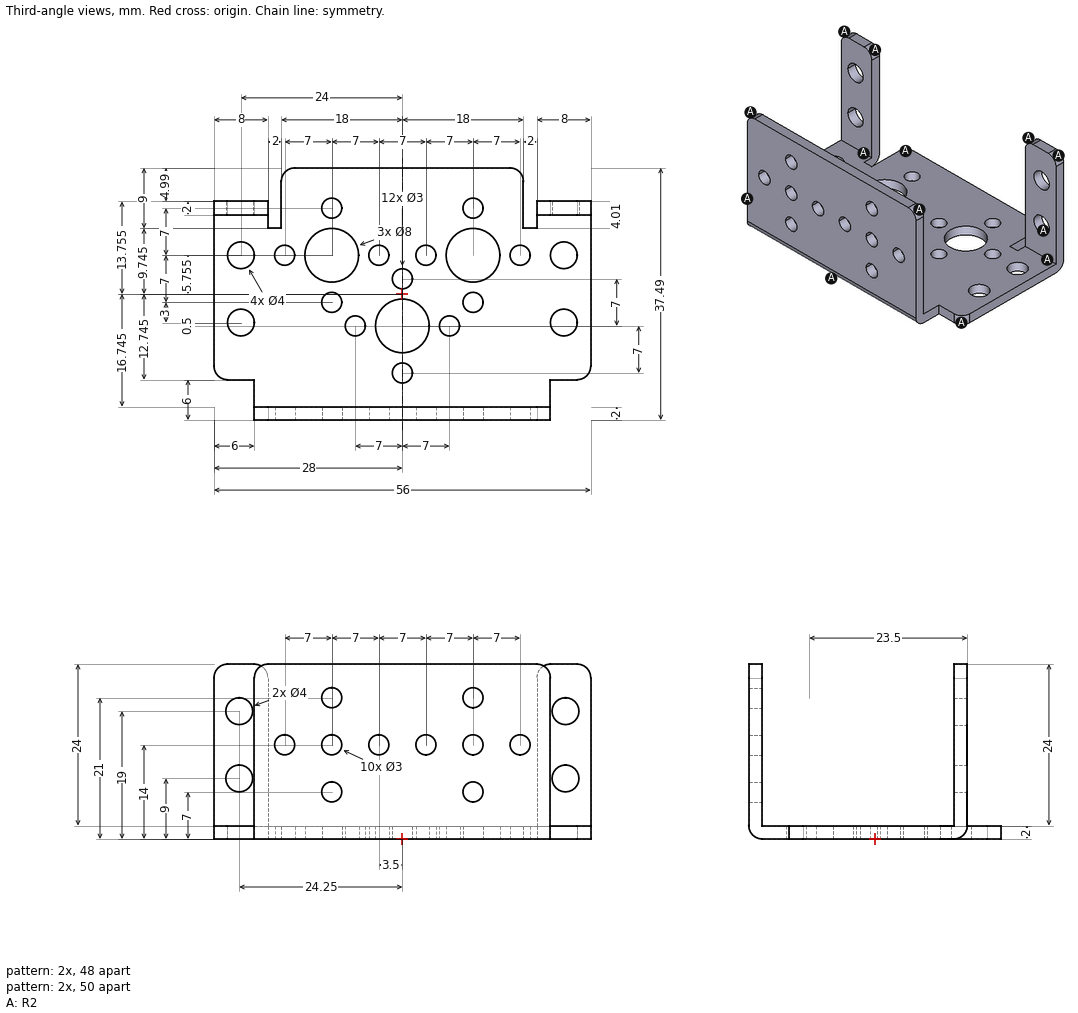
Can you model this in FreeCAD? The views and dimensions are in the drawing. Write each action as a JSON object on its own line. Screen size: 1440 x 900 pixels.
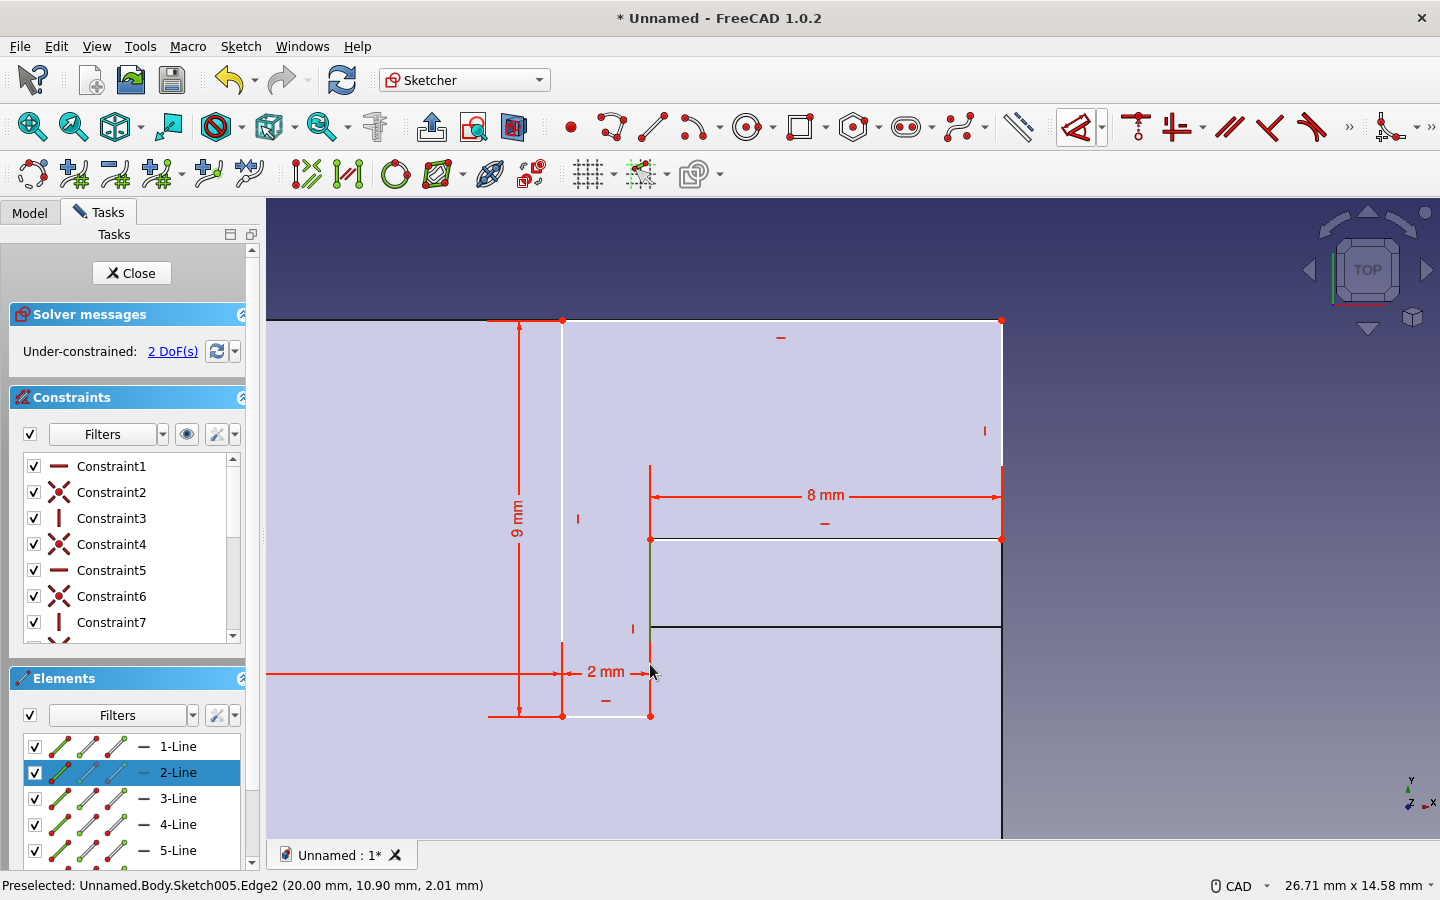
{"action": "key", "text": "i"}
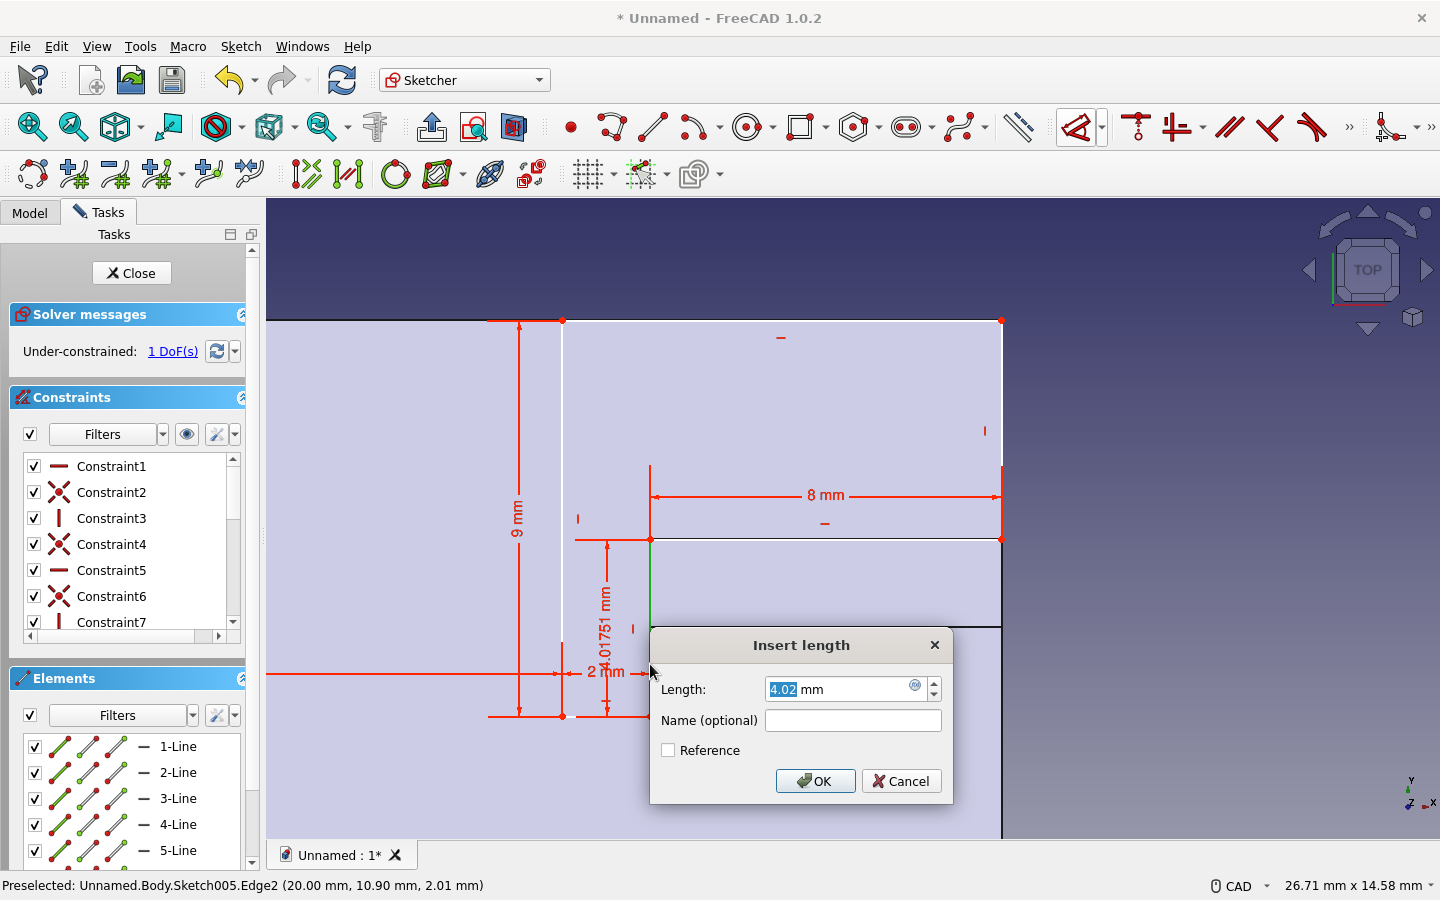
{"action": "type", "text": "4.01"}
{"action": "key", "text": "Return"}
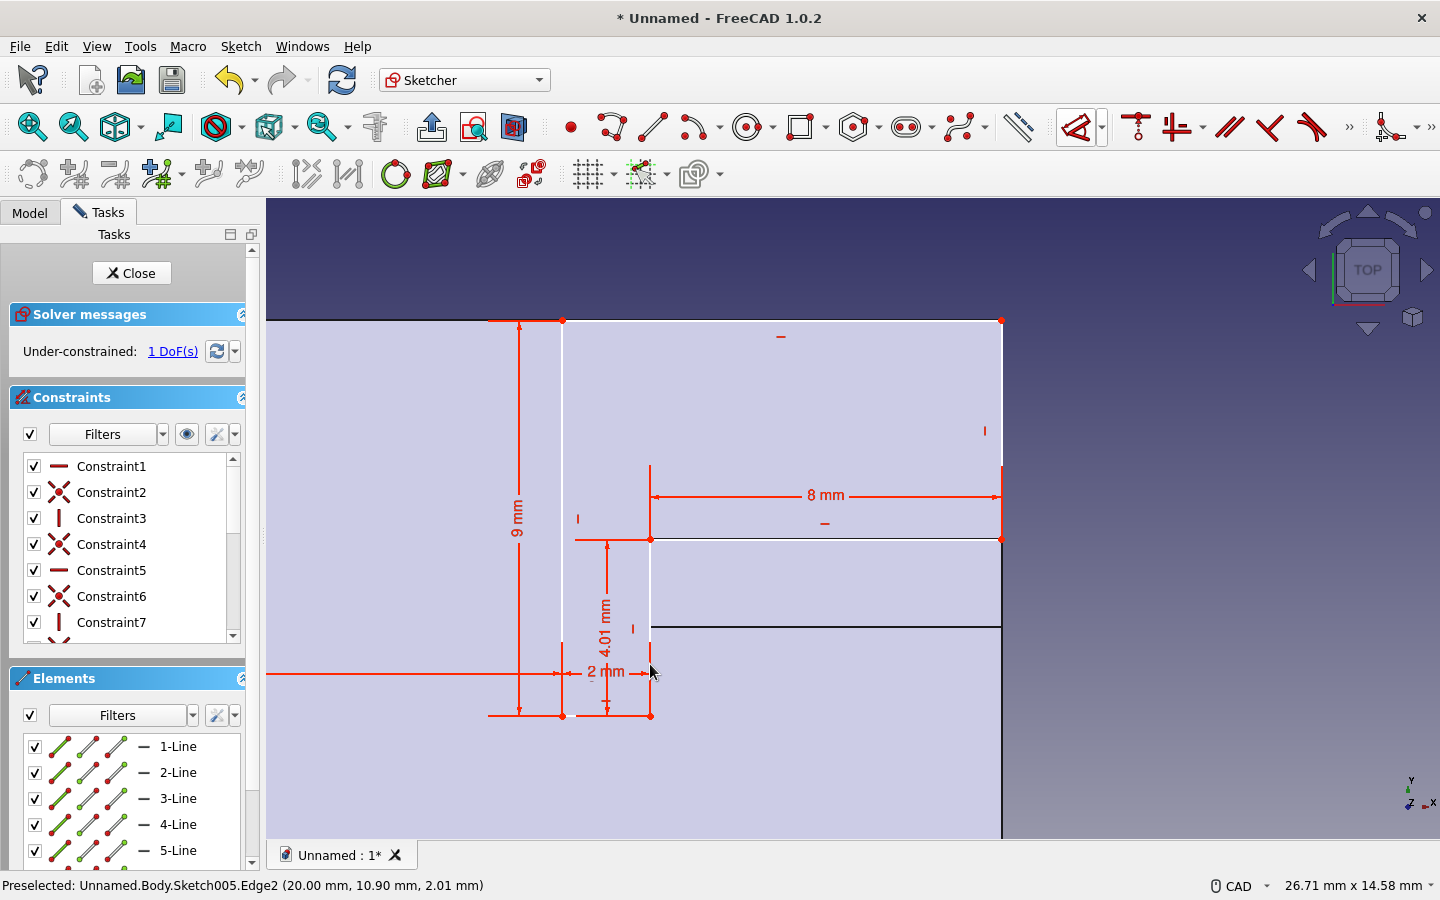
{"action": "left_click", "coordinate": [562, 716]}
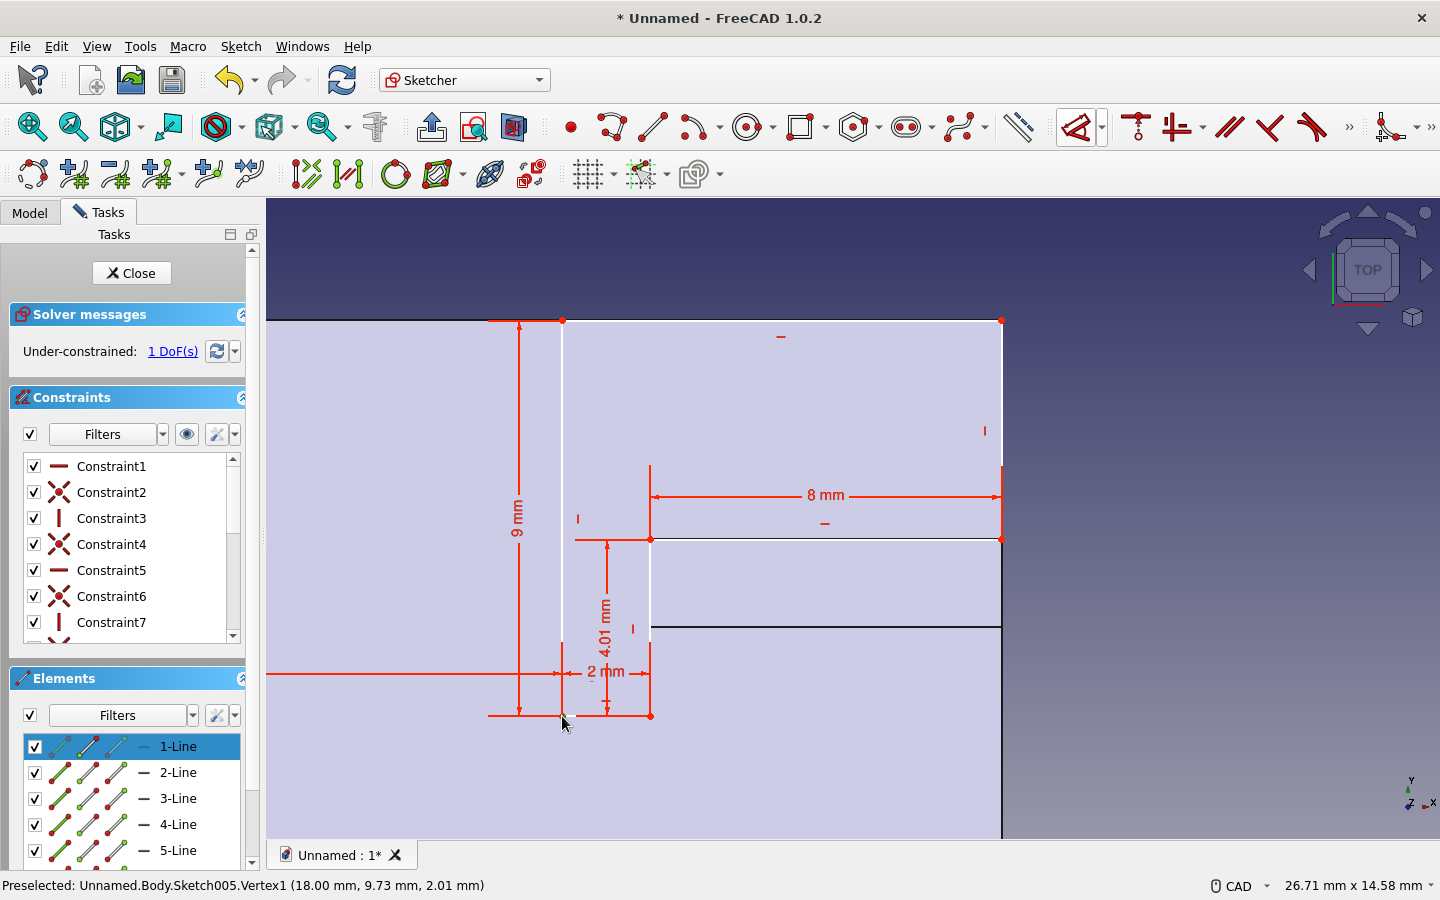
{"action": "key", "text": "i"}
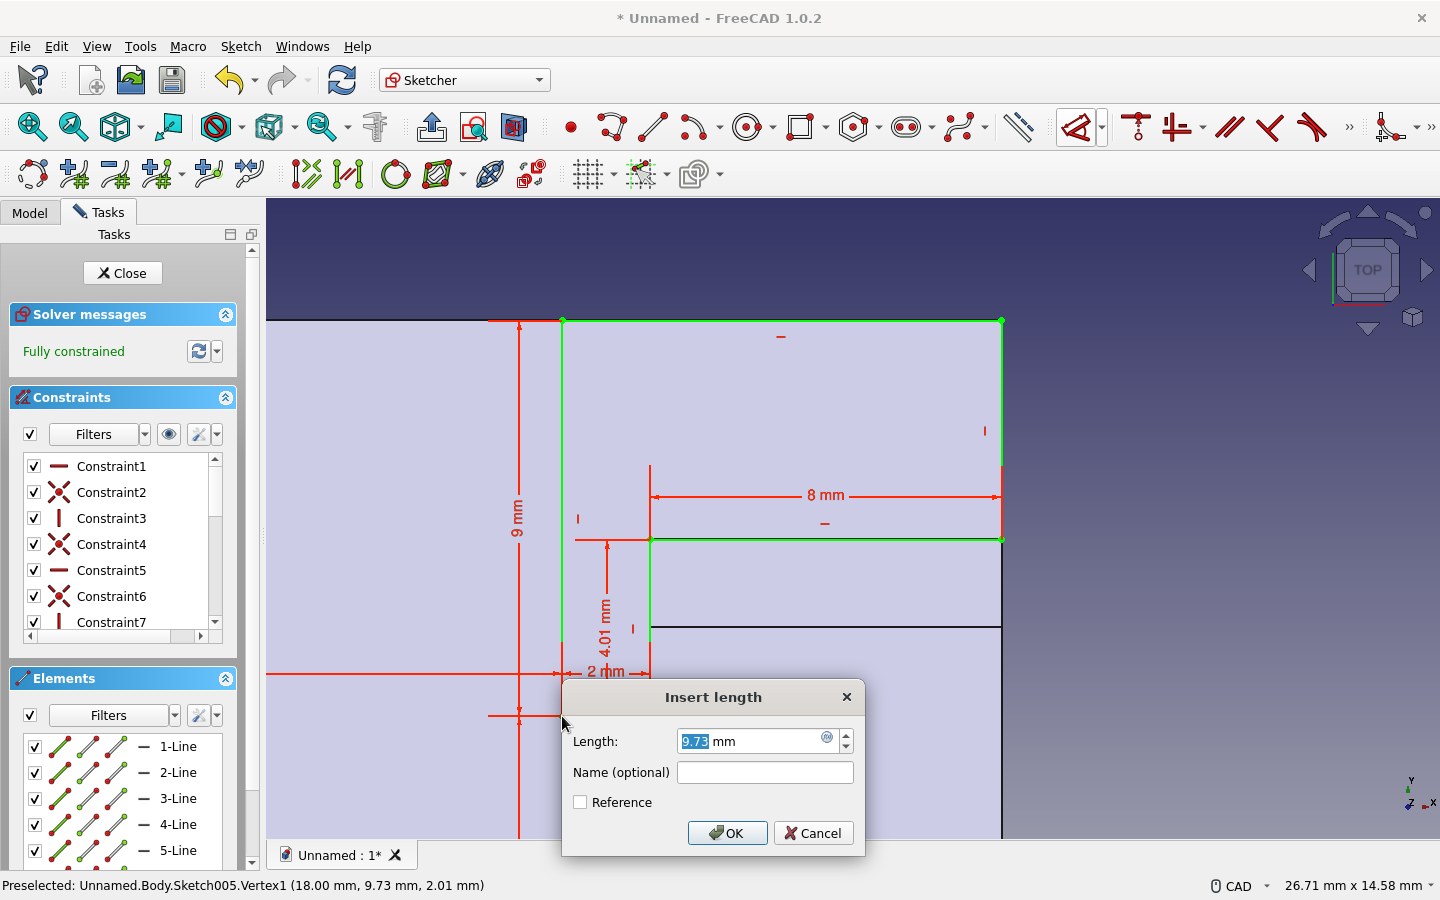
{"action": "type", "text": "9.745"}
{"action": "key", "text": "Return"}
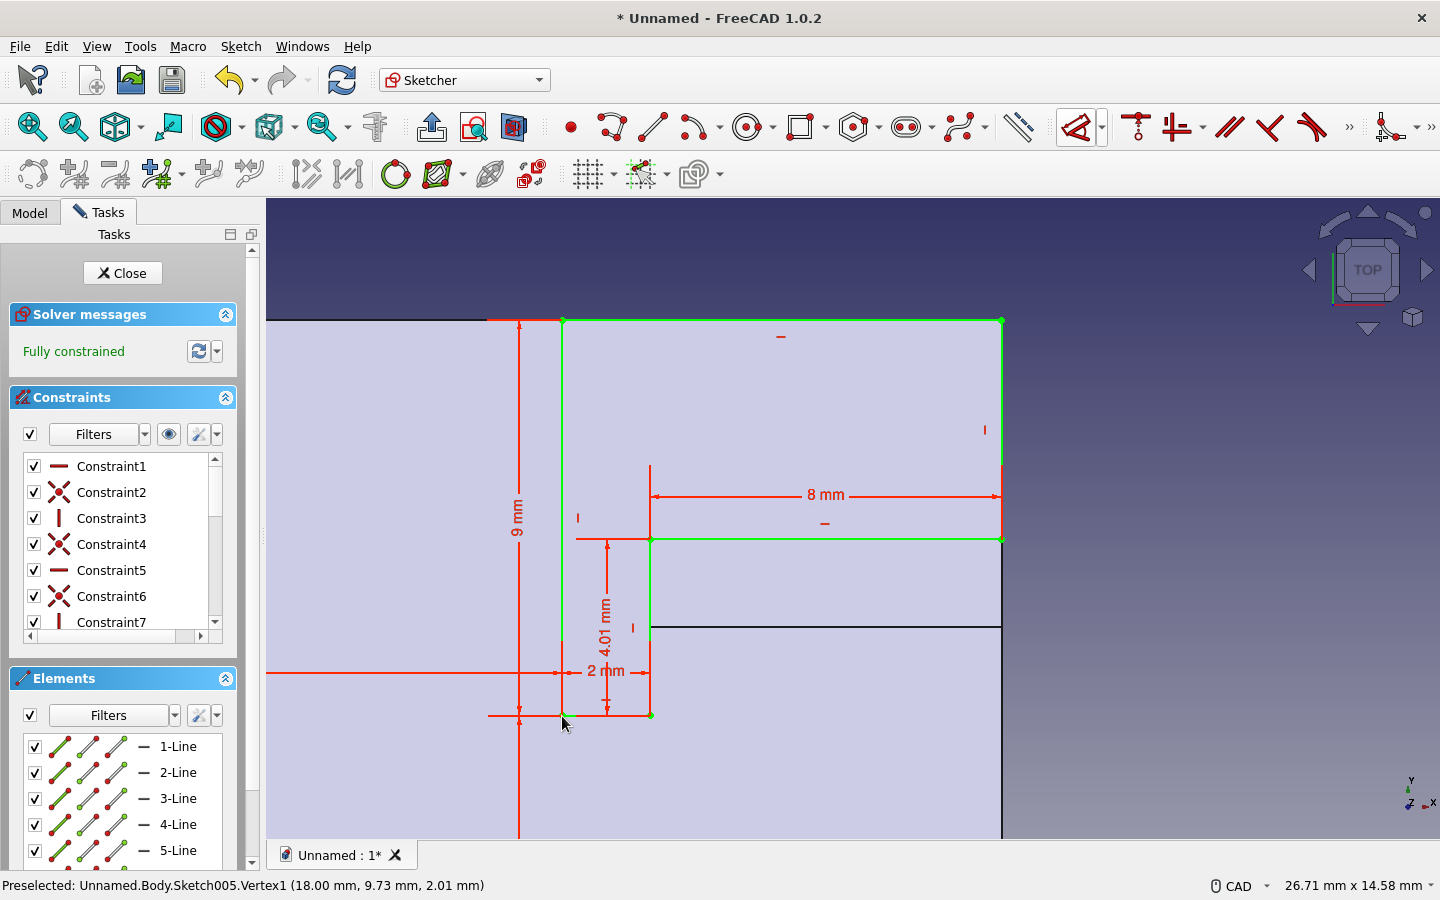
{"action": "left_click", "coordinate": [123, 273]}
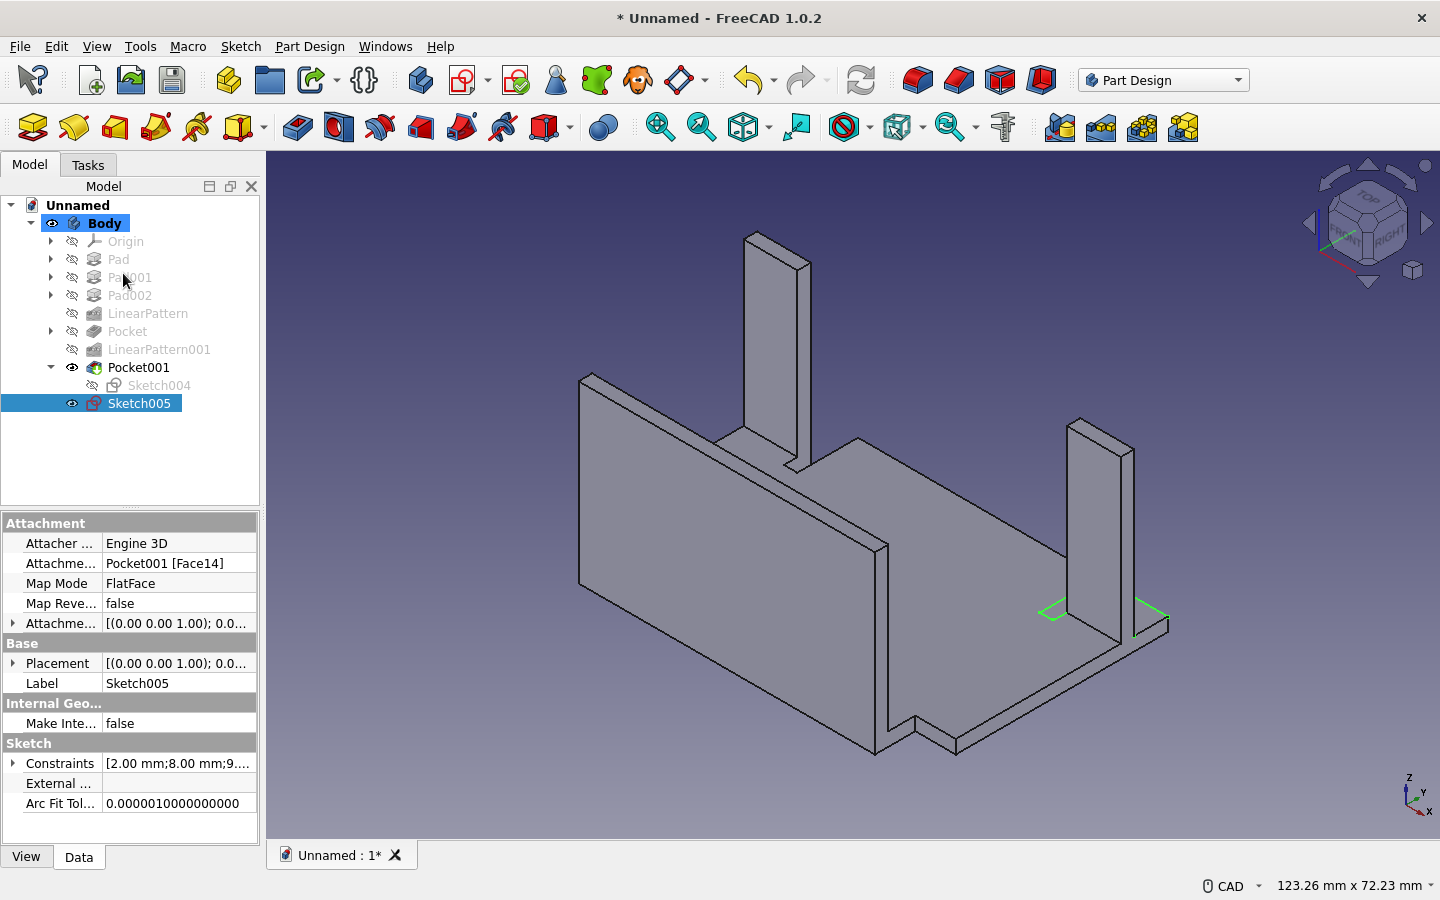
{"action": "left_click", "coordinate": [298, 128]}